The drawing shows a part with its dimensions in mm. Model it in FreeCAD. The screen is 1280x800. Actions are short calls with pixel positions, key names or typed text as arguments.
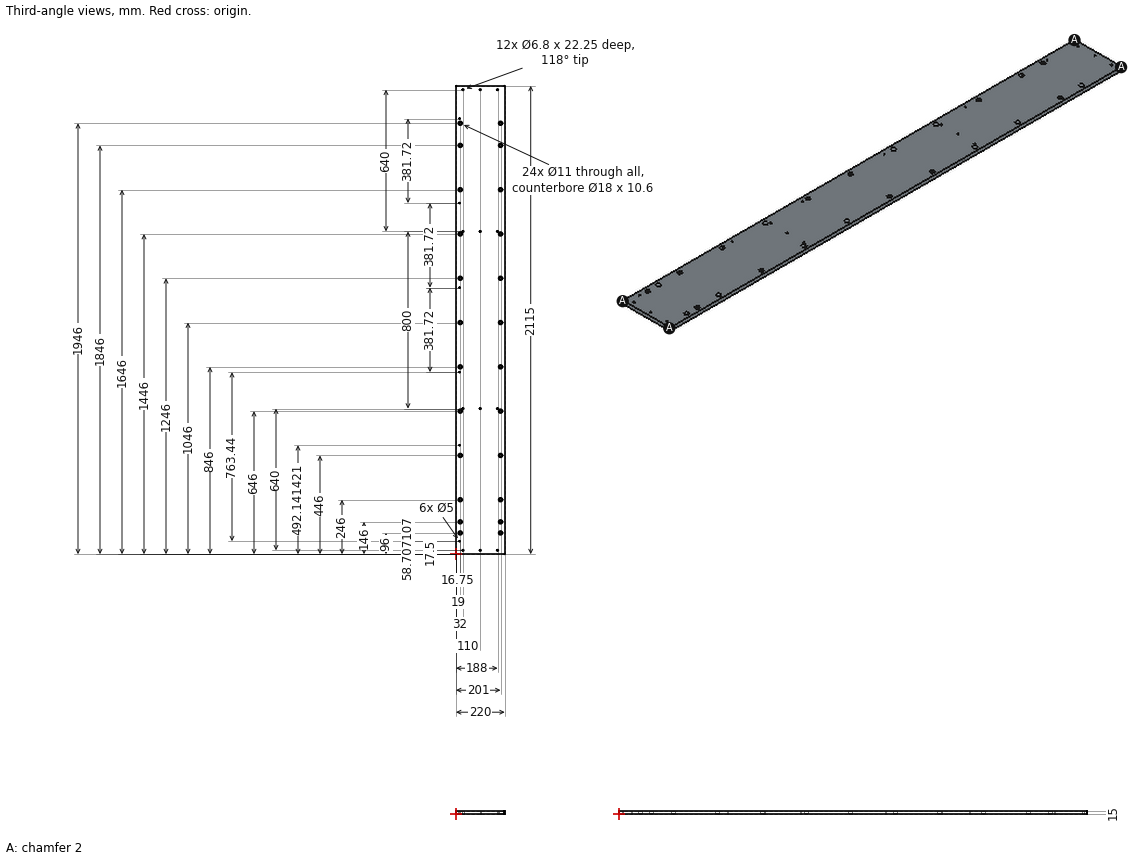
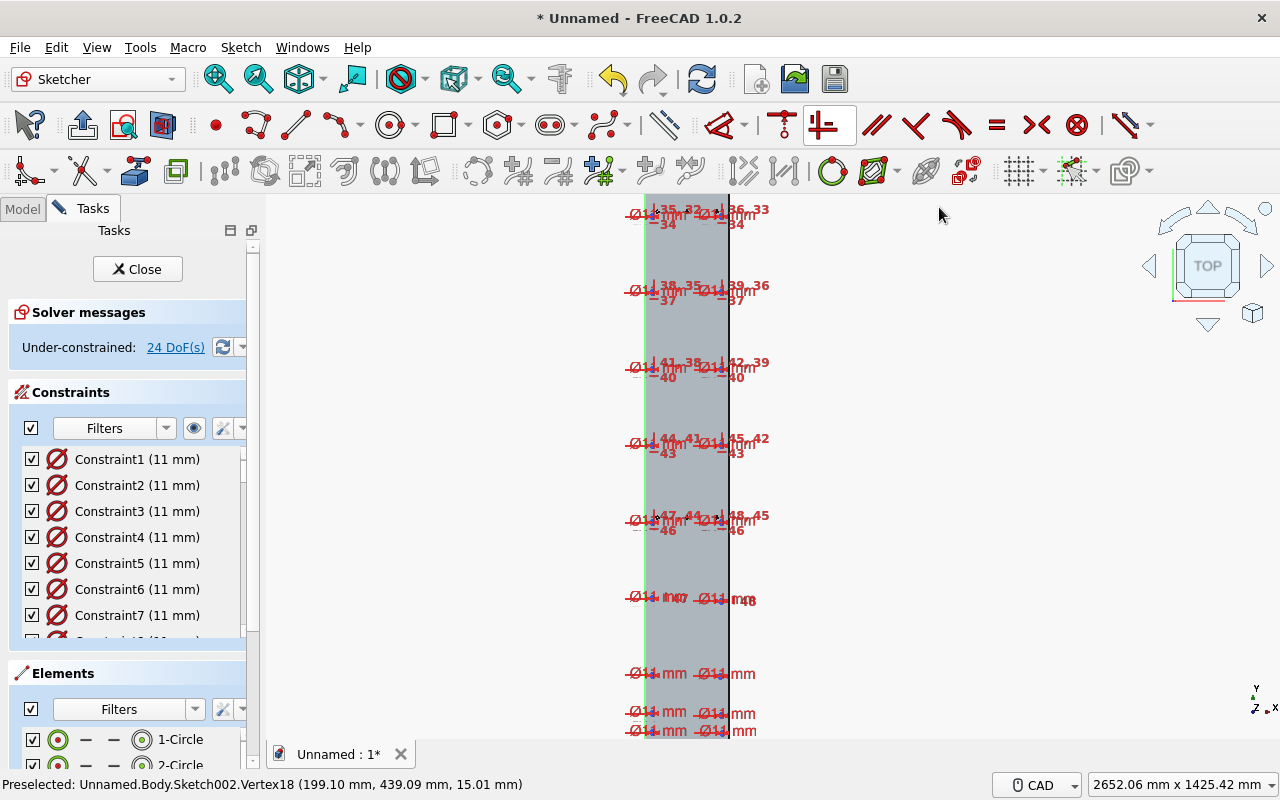
click(652, 599)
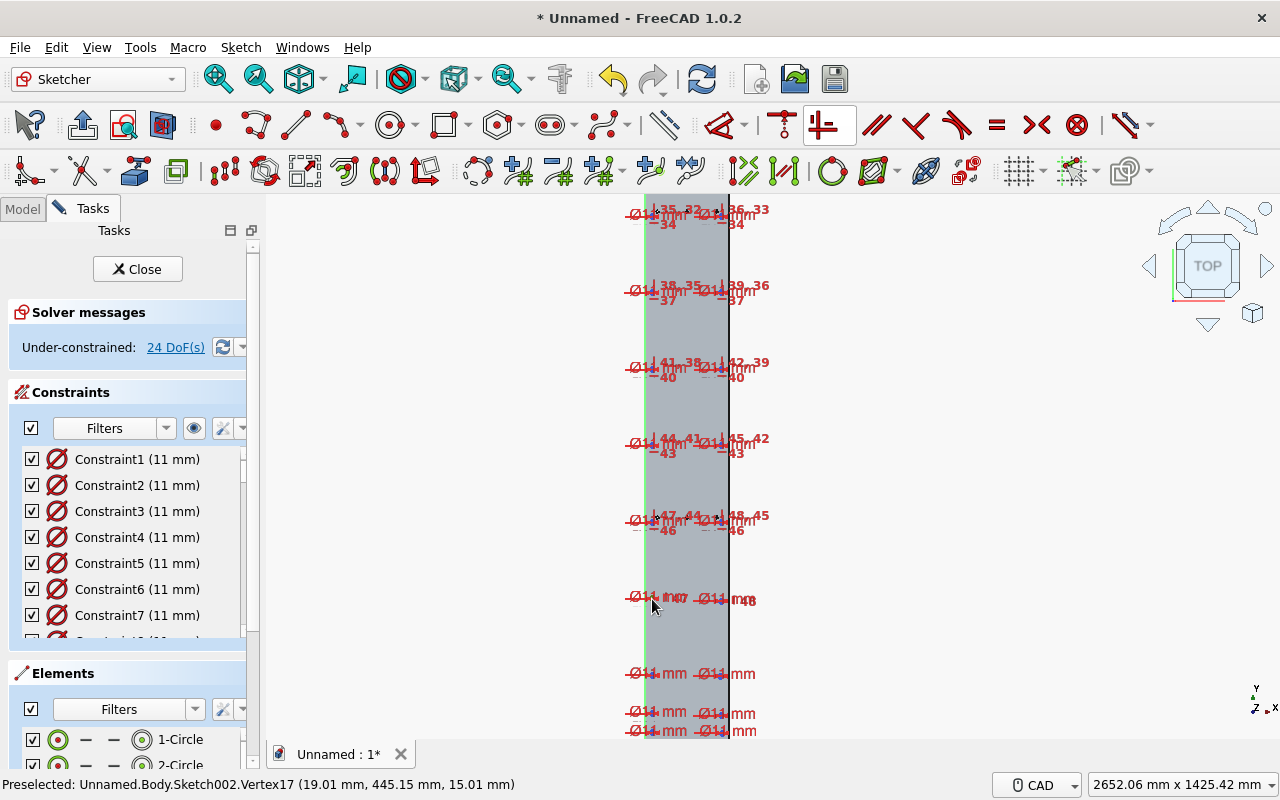
click(721, 601)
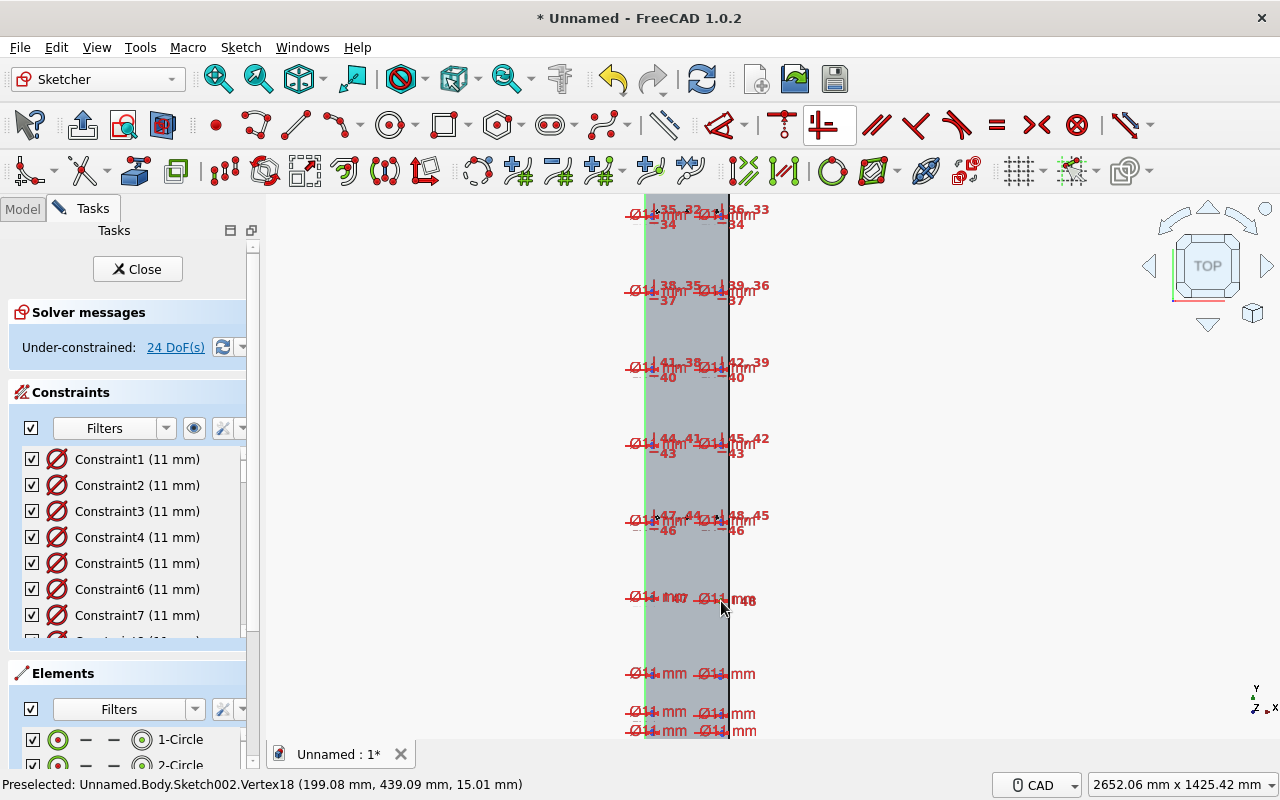
click(850, 126)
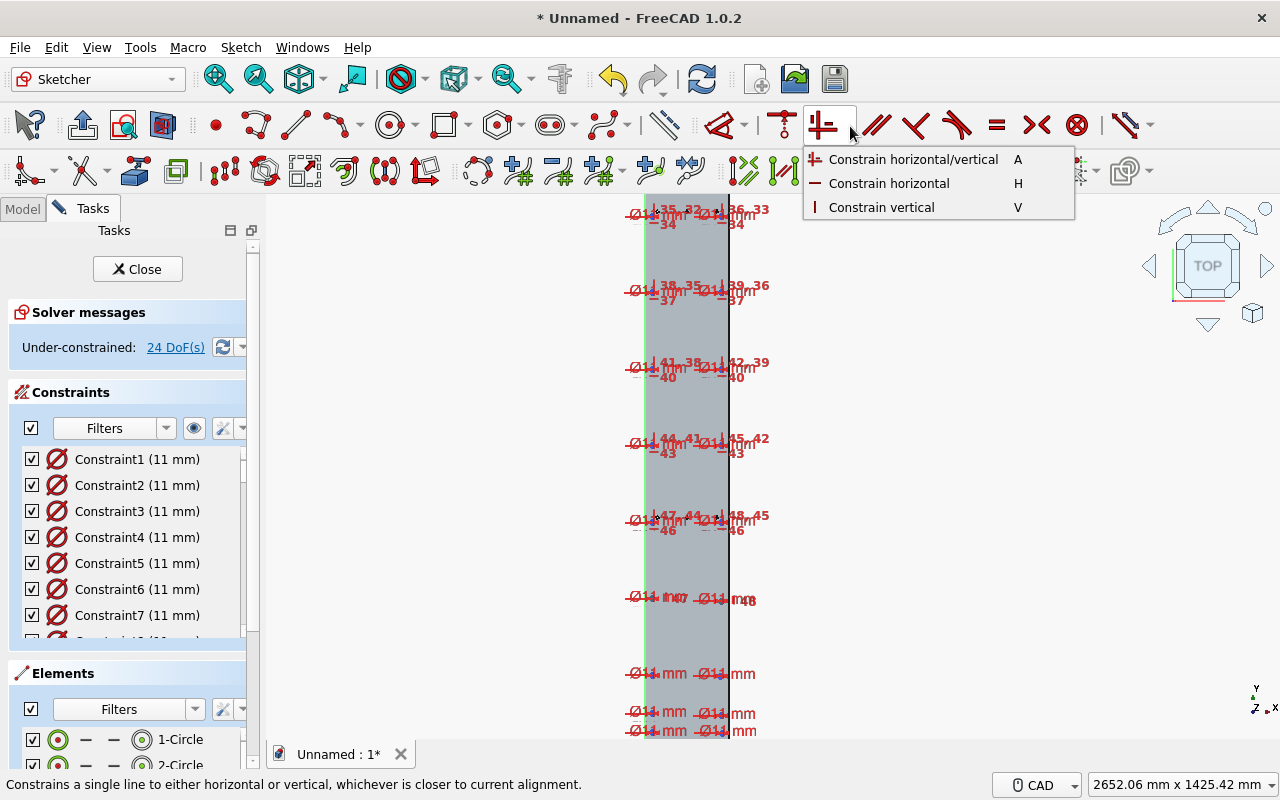
click(939, 183)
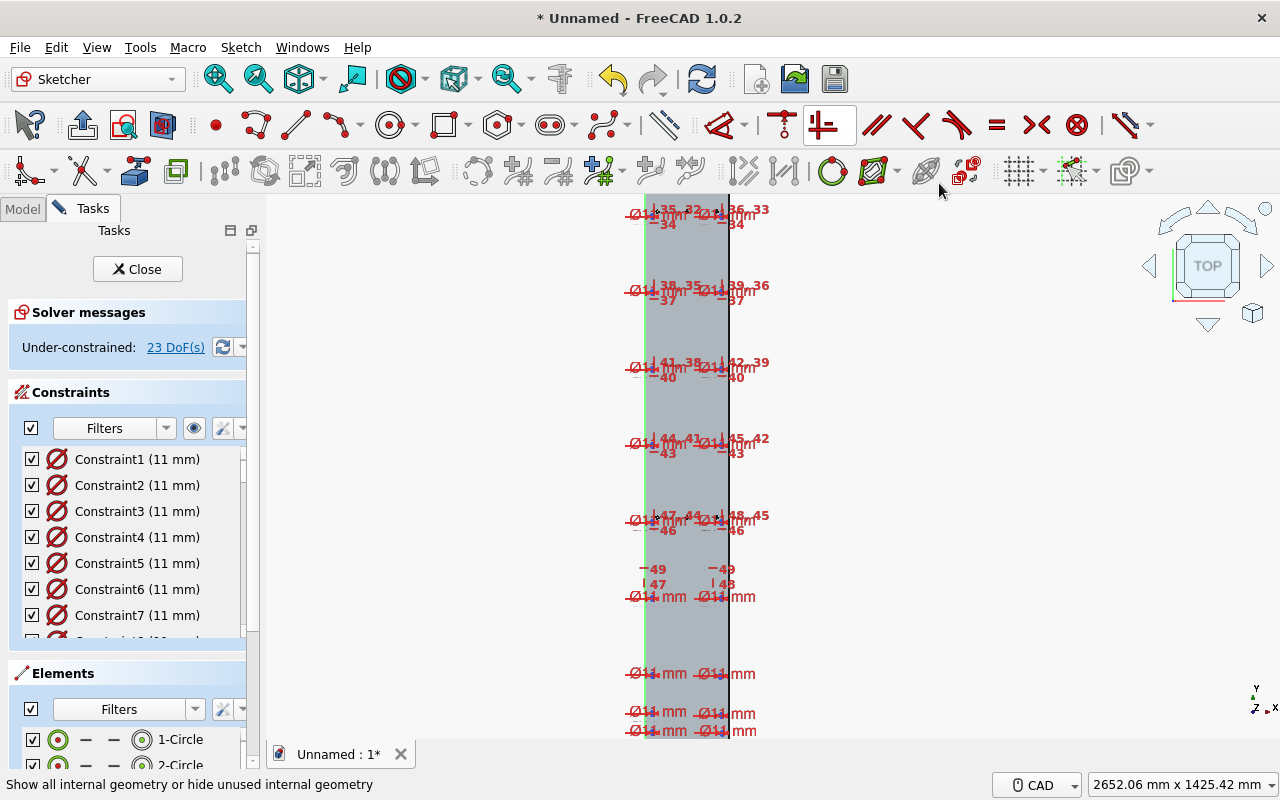
click(652, 599)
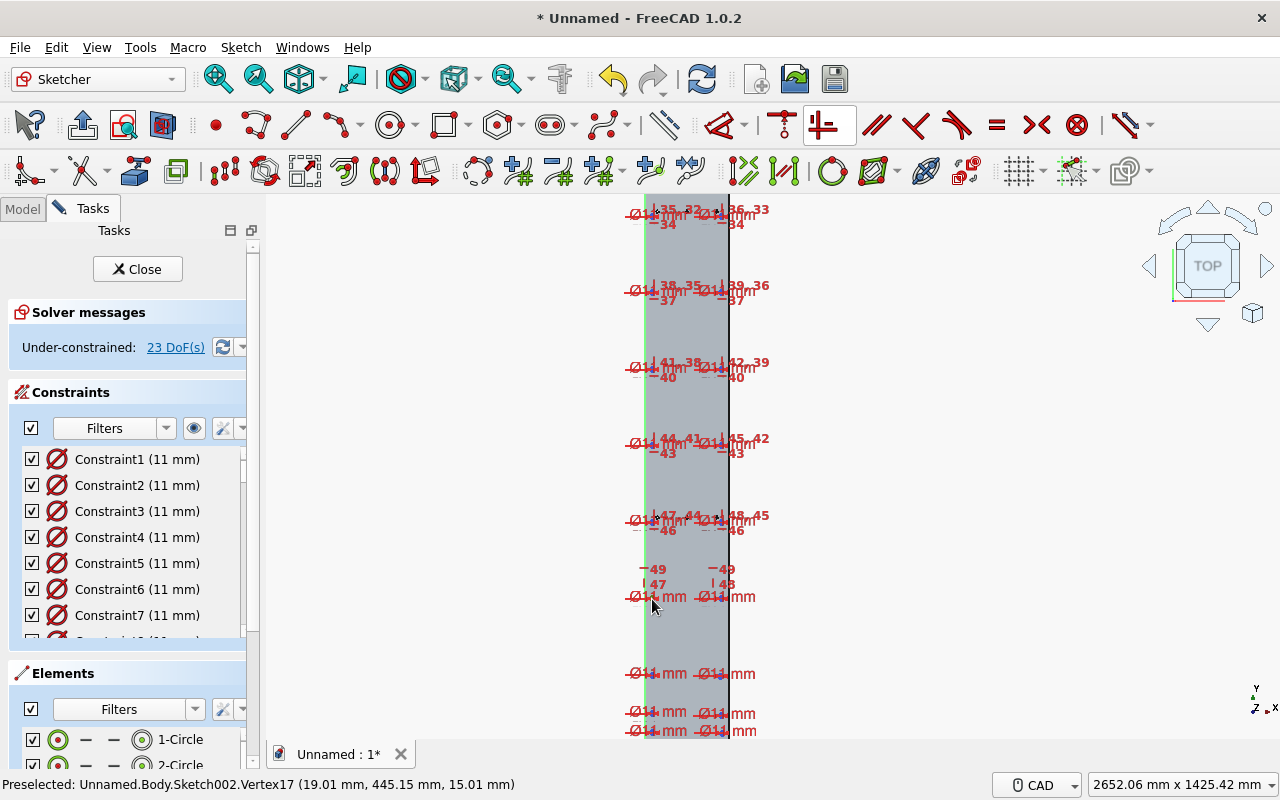
click(652, 675)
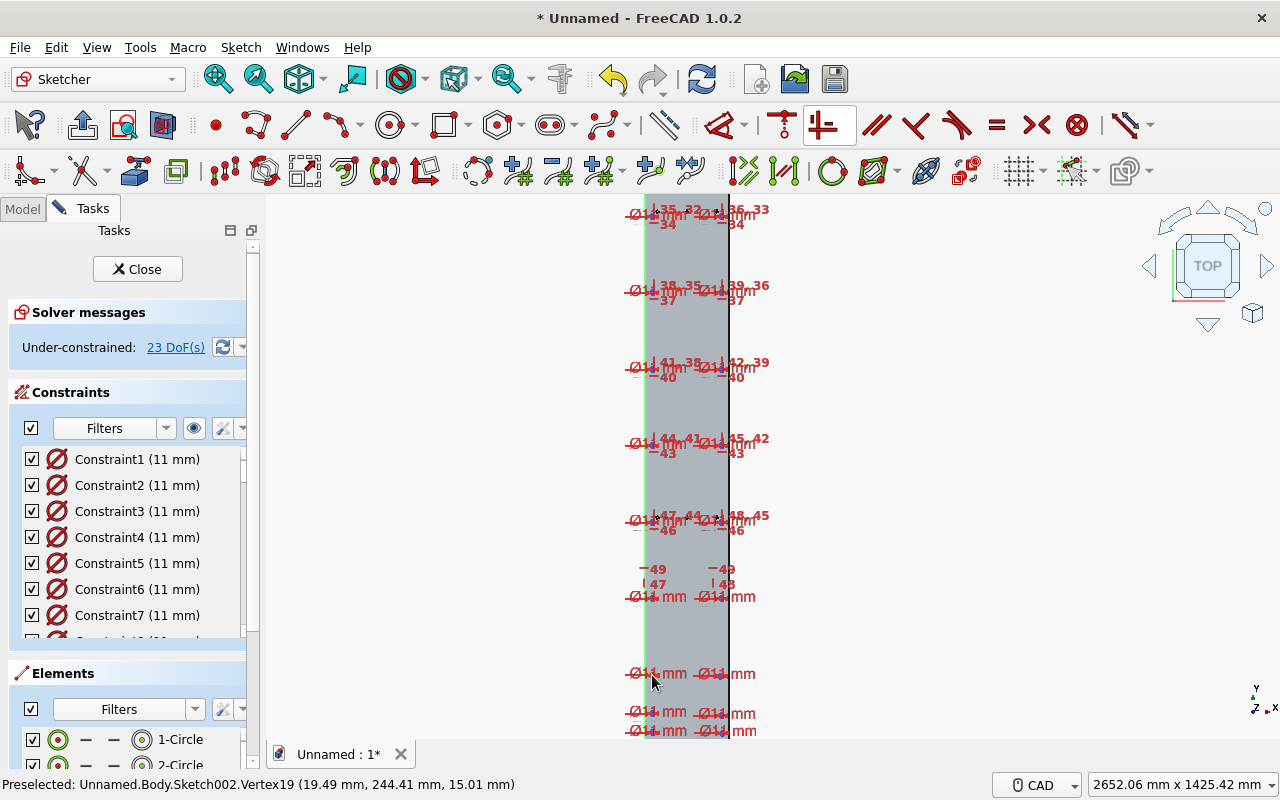
click(850, 126)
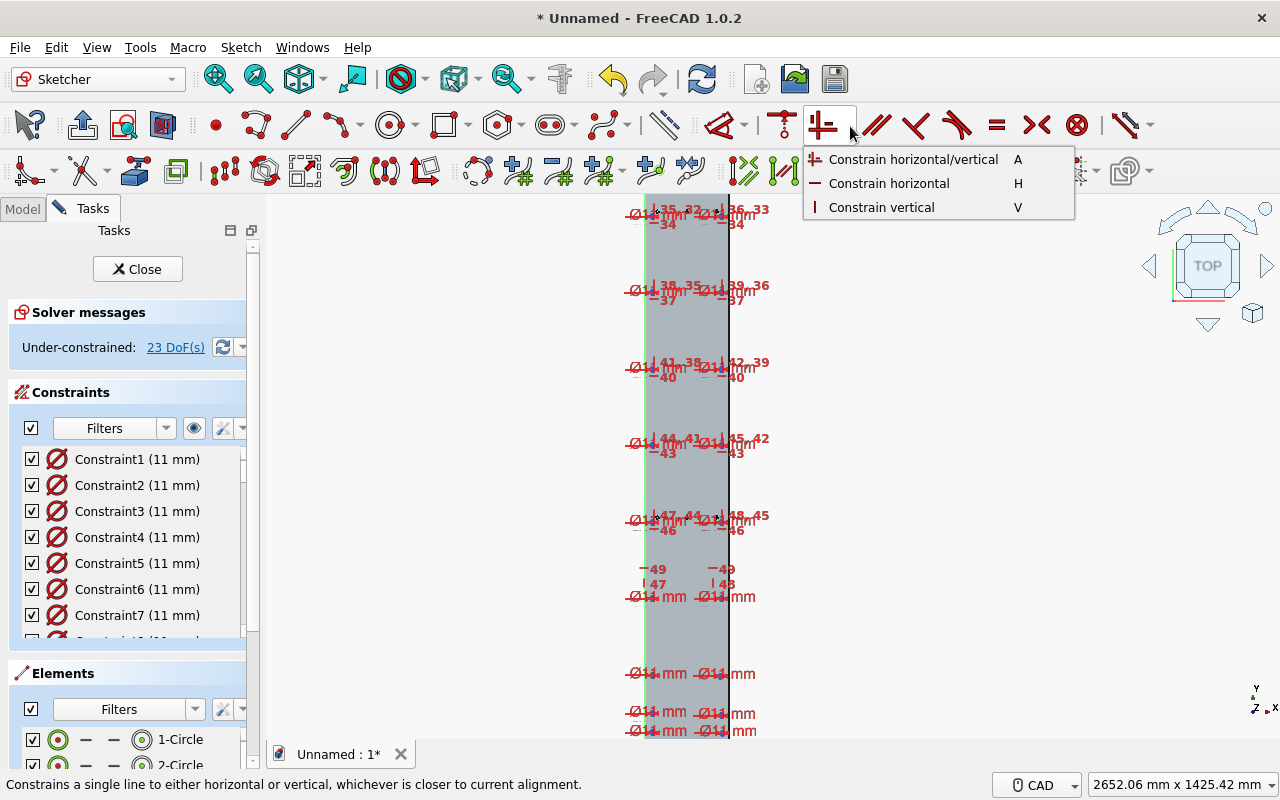
click(939, 207)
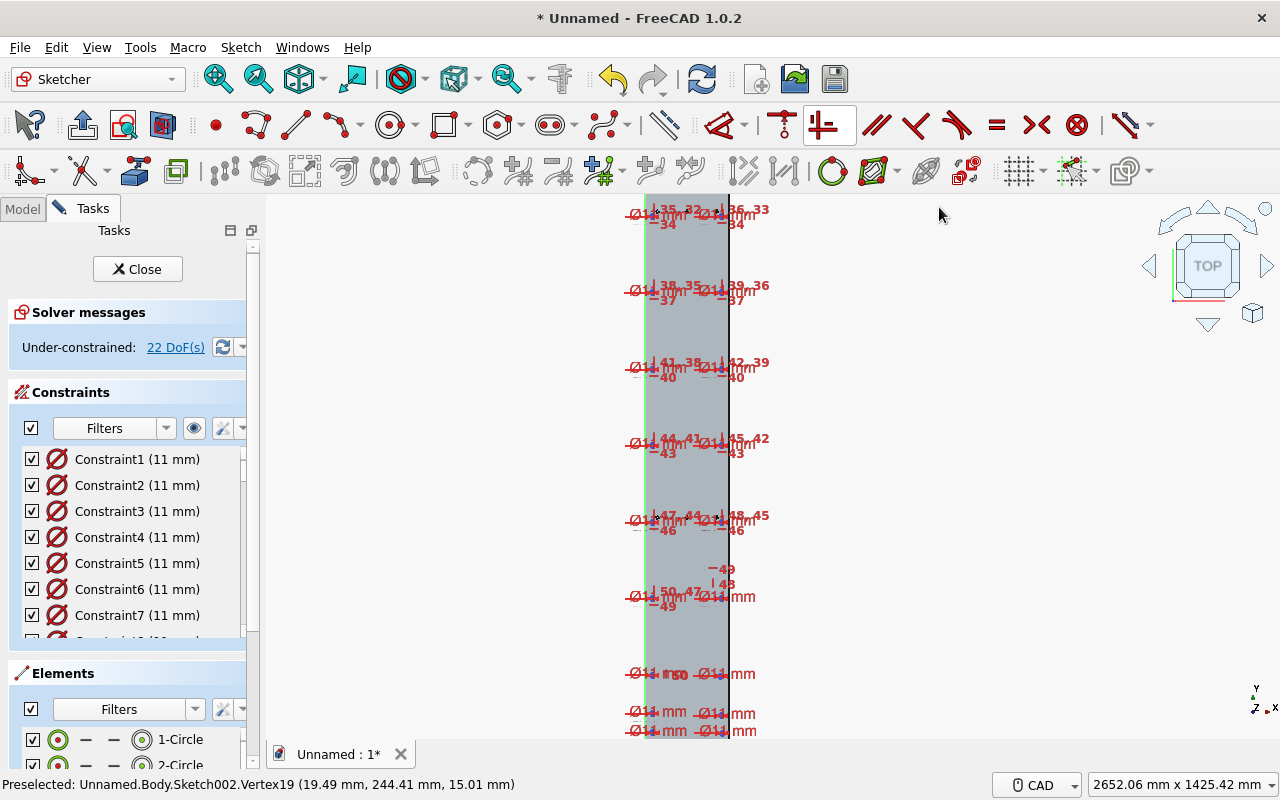
click(721, 599)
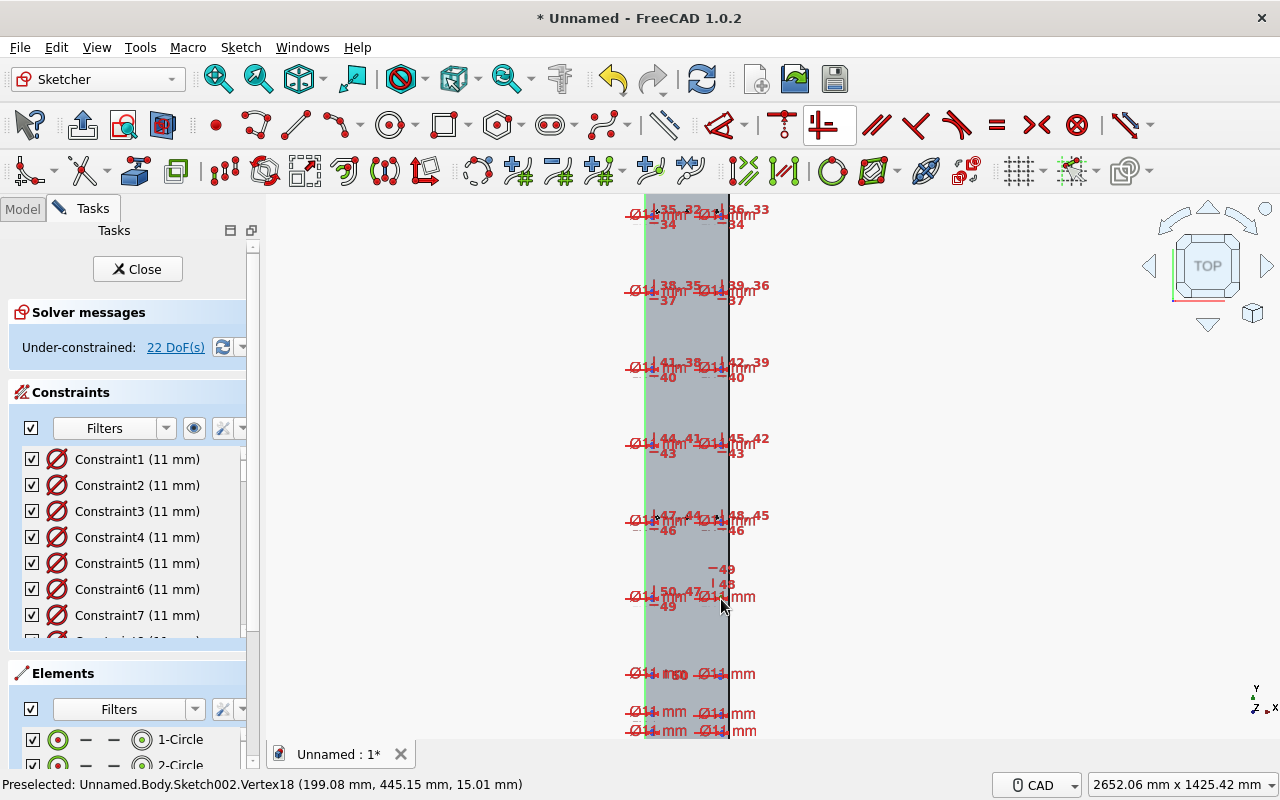
click(721, 676)